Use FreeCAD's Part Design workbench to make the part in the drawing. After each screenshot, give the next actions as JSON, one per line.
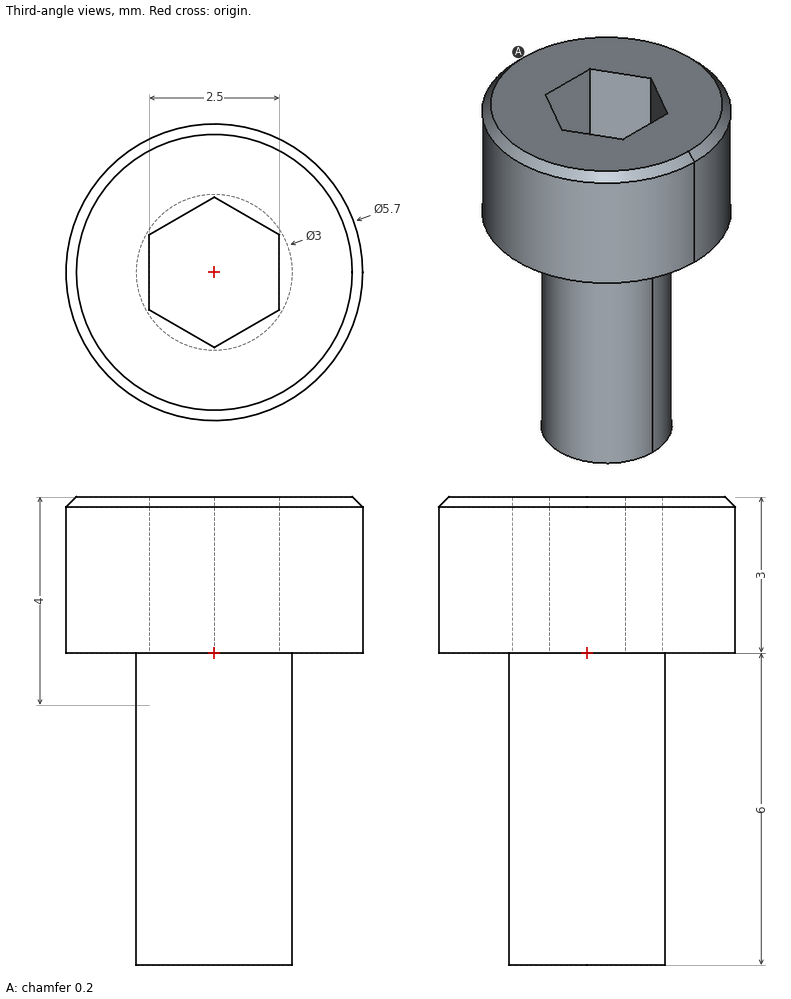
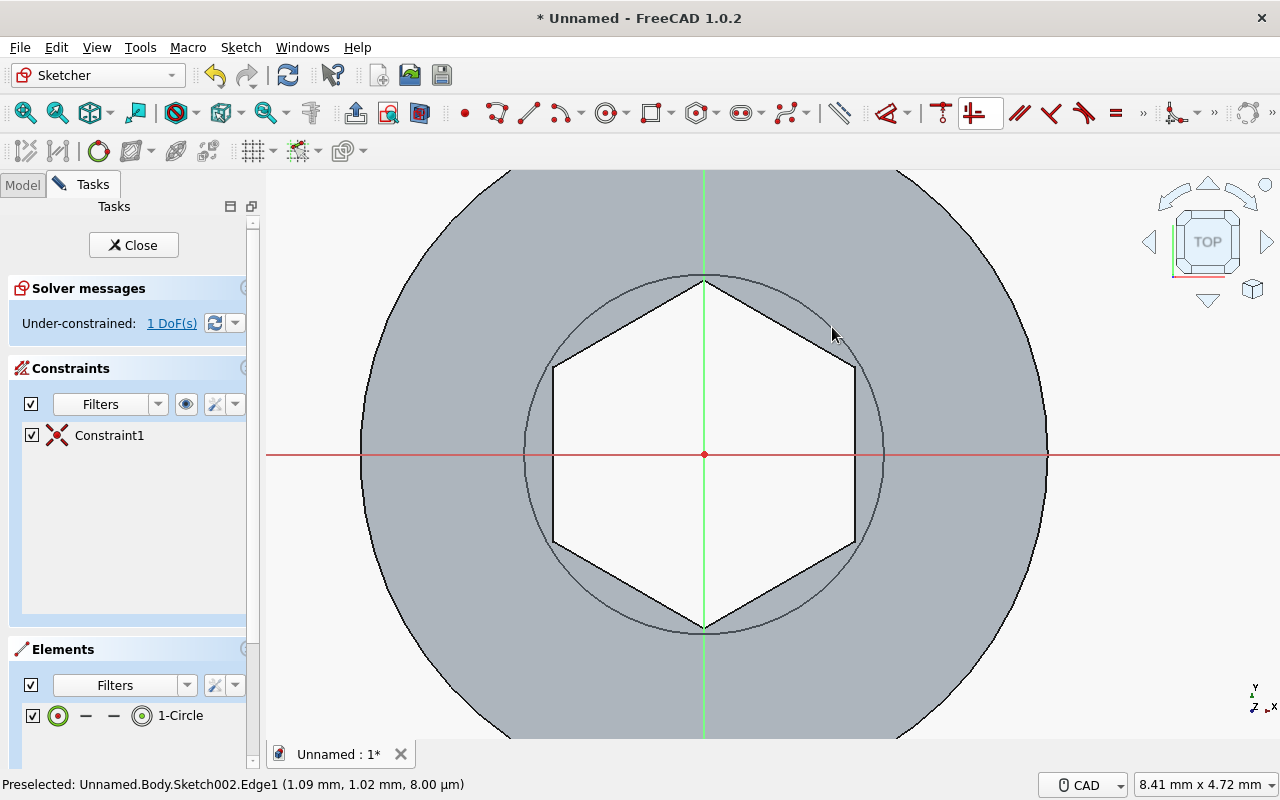
{"action": "left_click", "coordinate": [886, 114]}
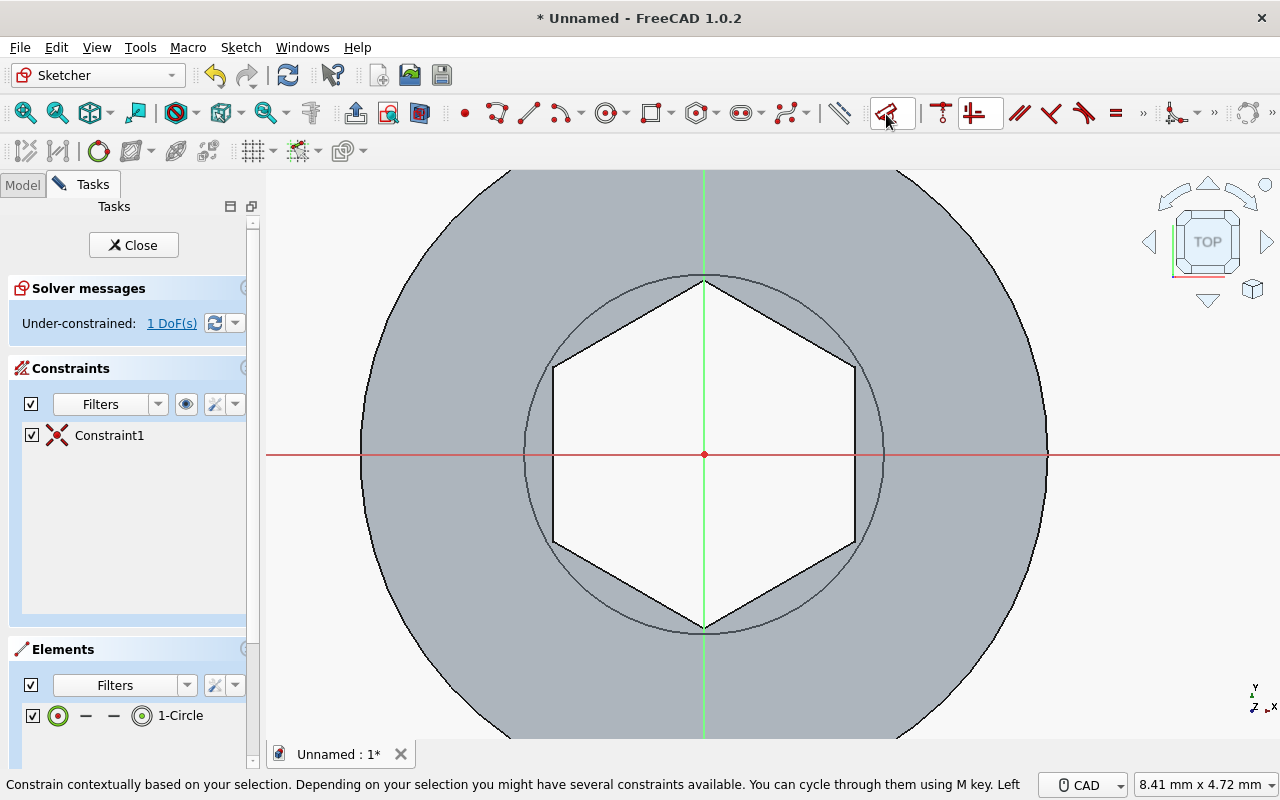
{"action": "left_click", "coordinate": [831, 327]}
{"action": "left_click", "coordinate": [854, 304]}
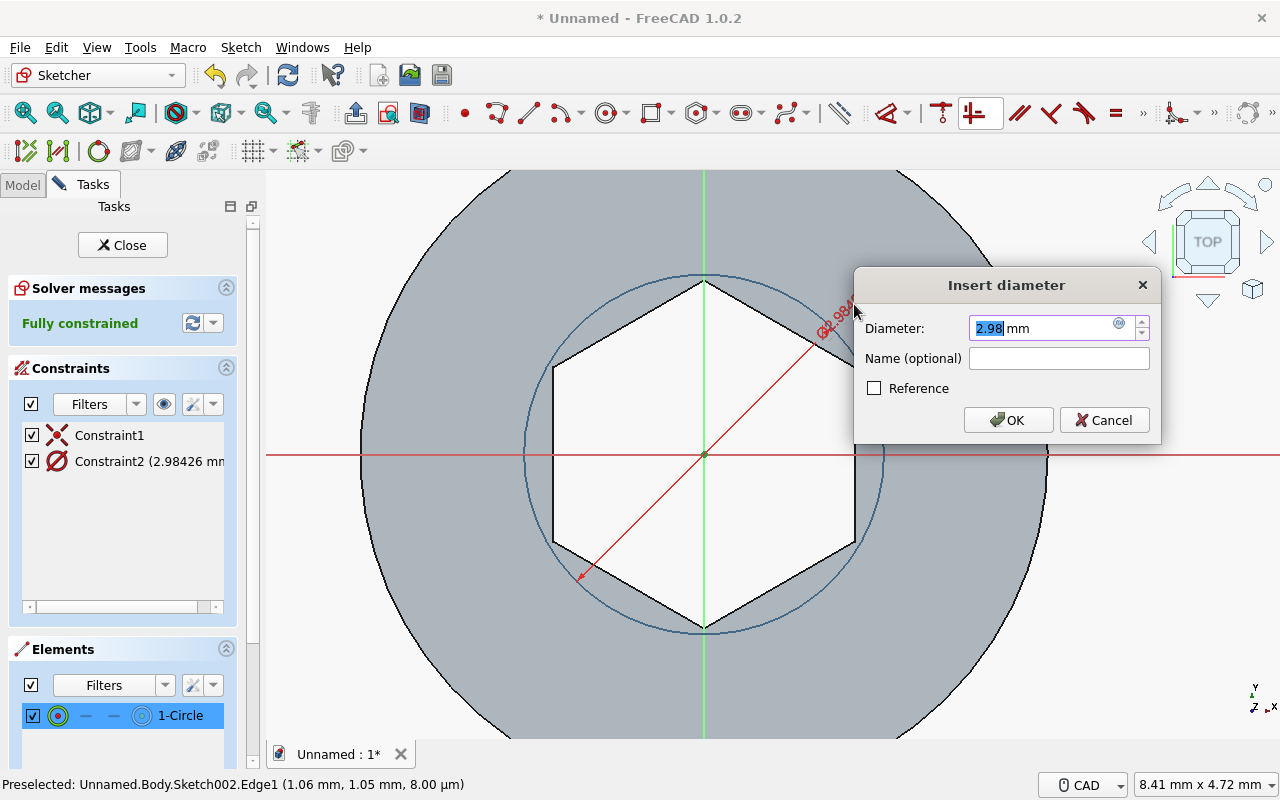
{"action": "type", "text": "3"}
{"action": "key", "text": "Return"}
{"action": "key", "text": "Escape"}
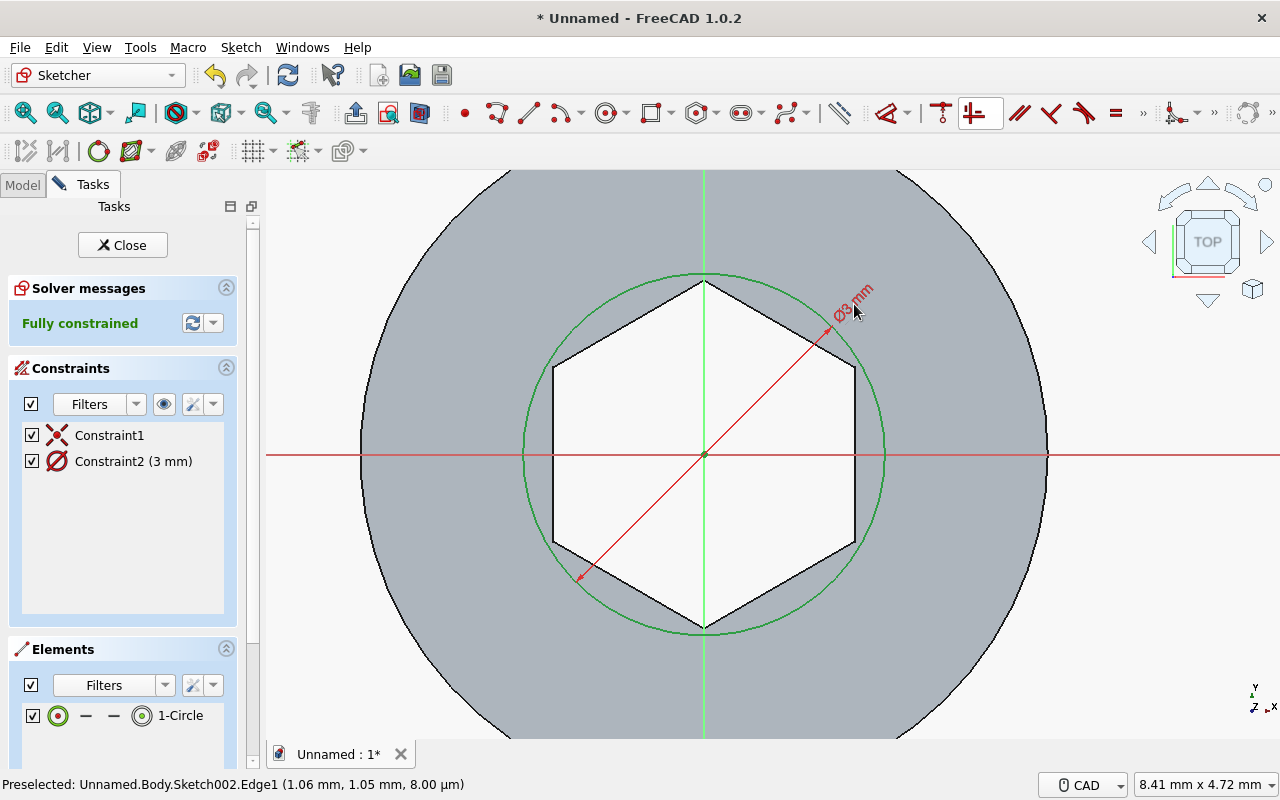
{"action": "left_click", "coordinate": [123, 245]}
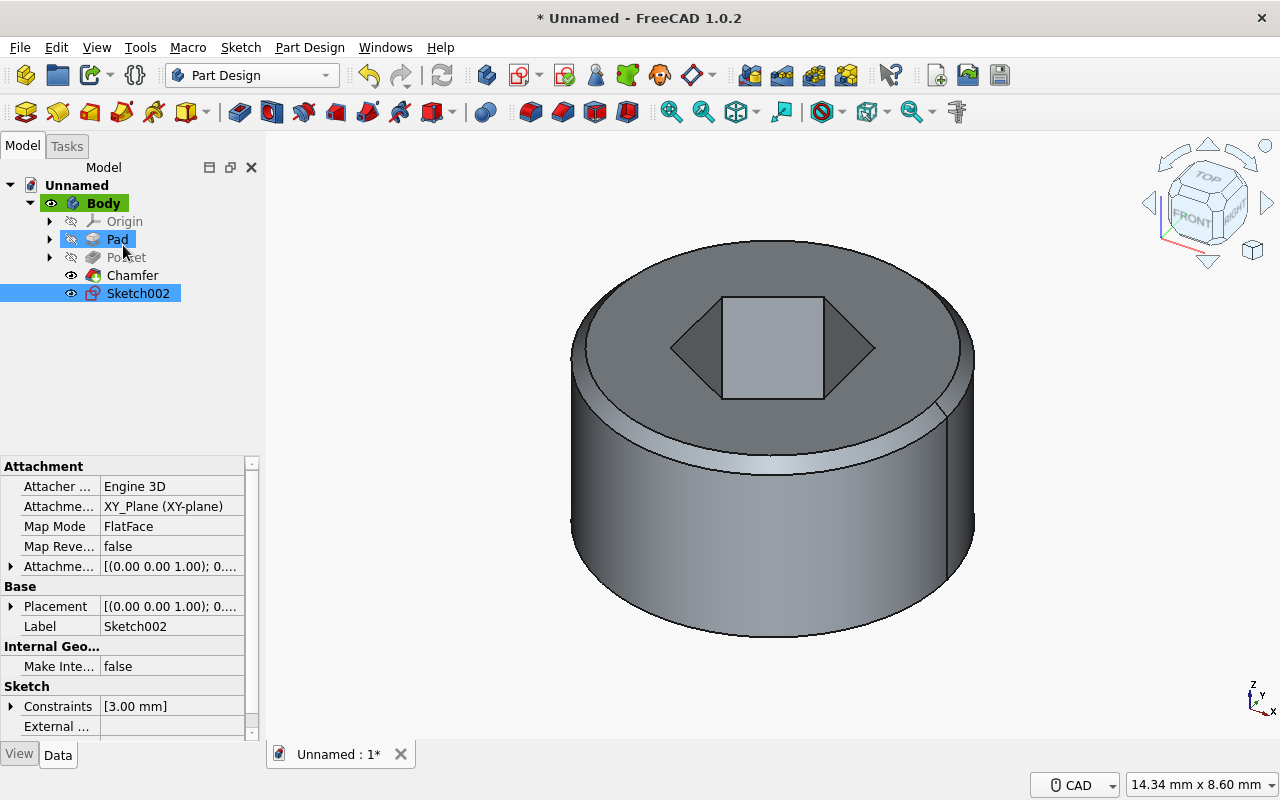
{"action": "left_click", "coordinate": [26, 112]}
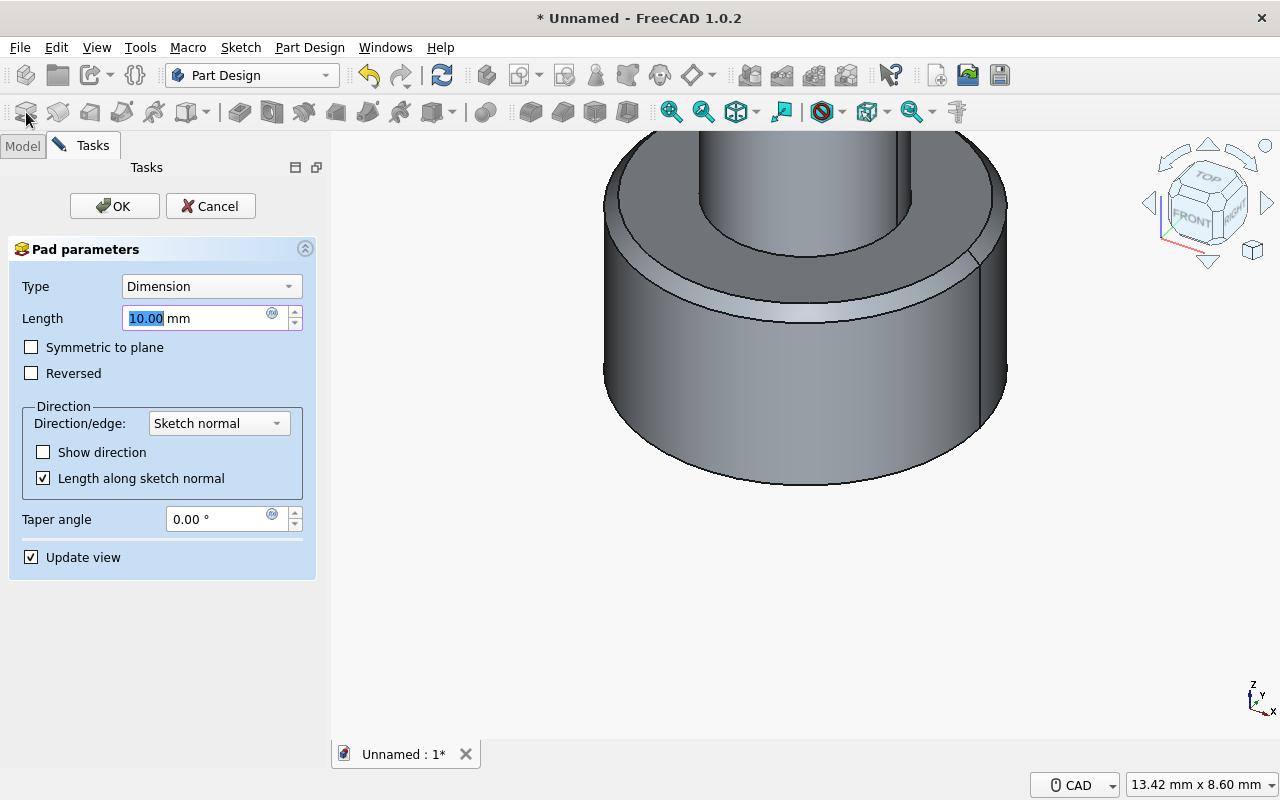
{"action": "type", "text": "6"}
{"action": "key", "text": "Tab"}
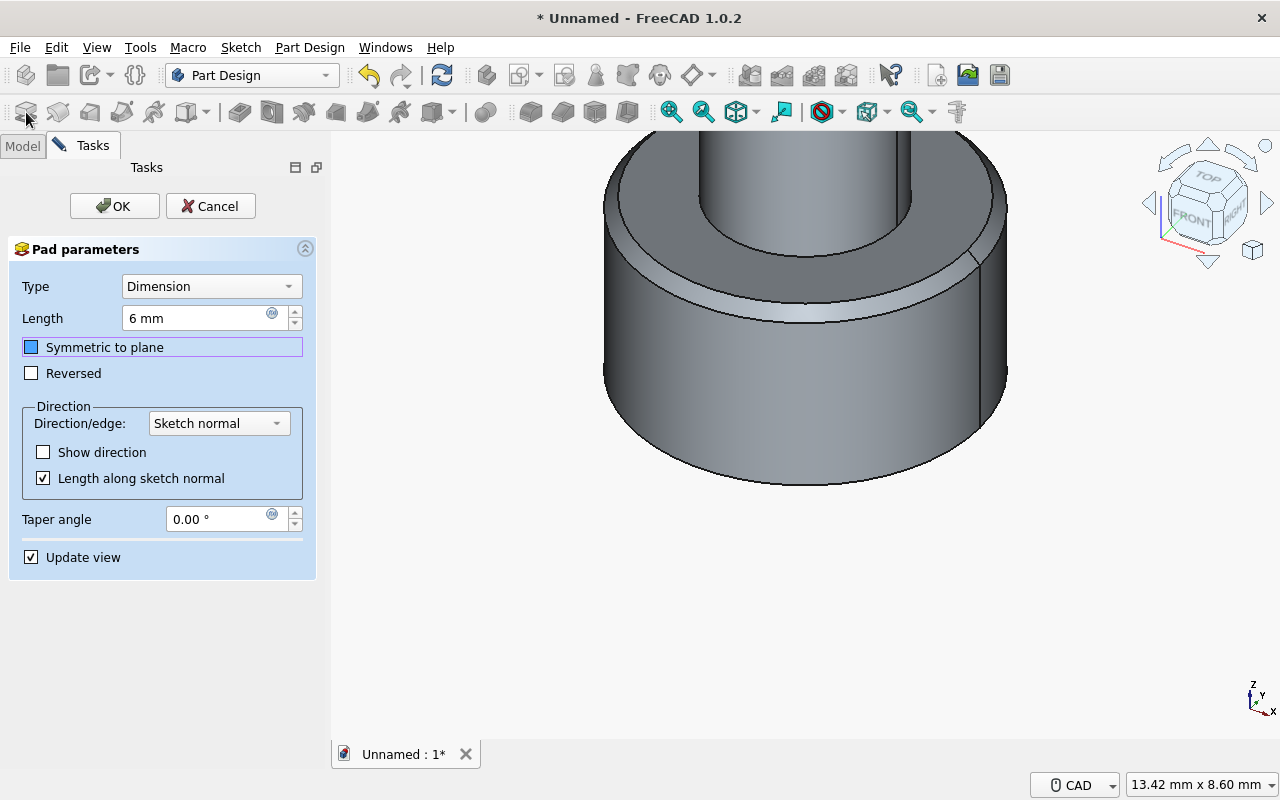
{"action": "left_click", "coordinate": [30, 373]}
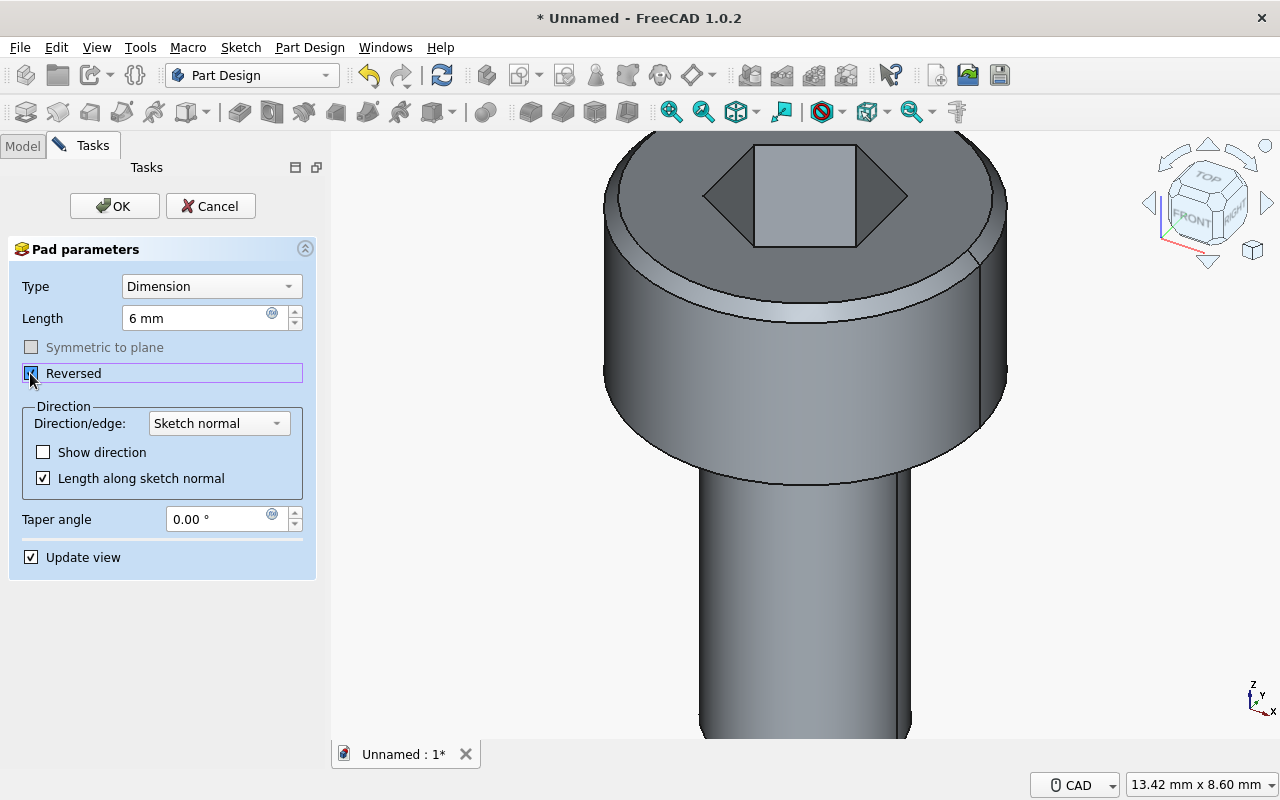
{"action": "left_click", "coordinate": [115, 206]}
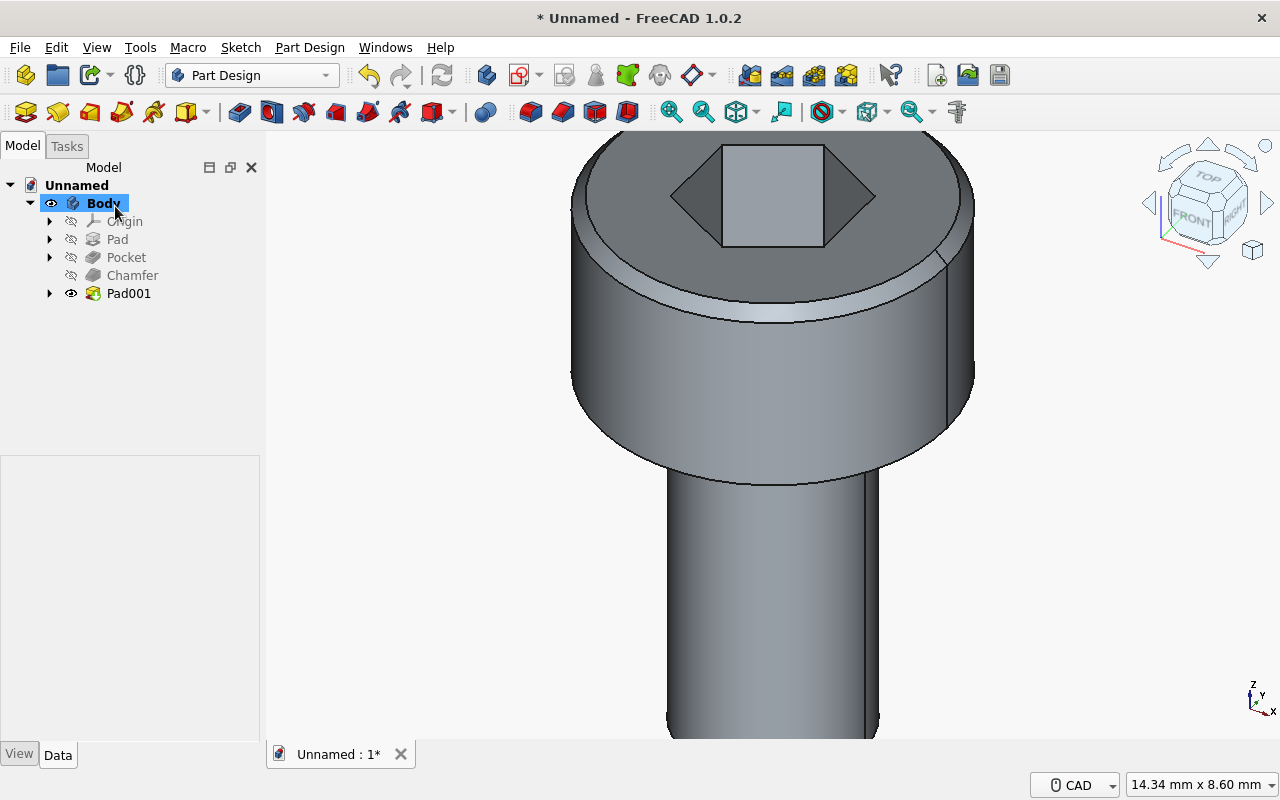
{"action": "key", "text": "0"}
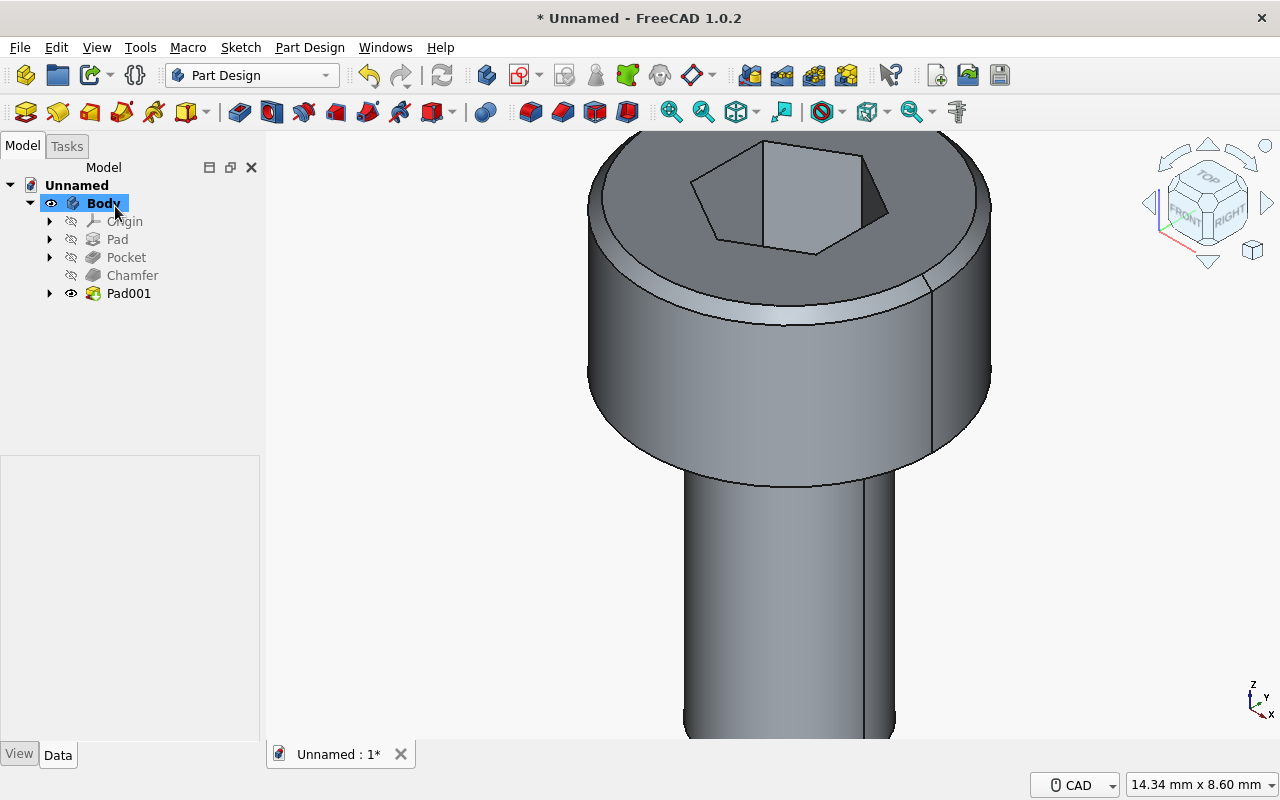
{"action": "left_click", "coordinate": [672, 112]}